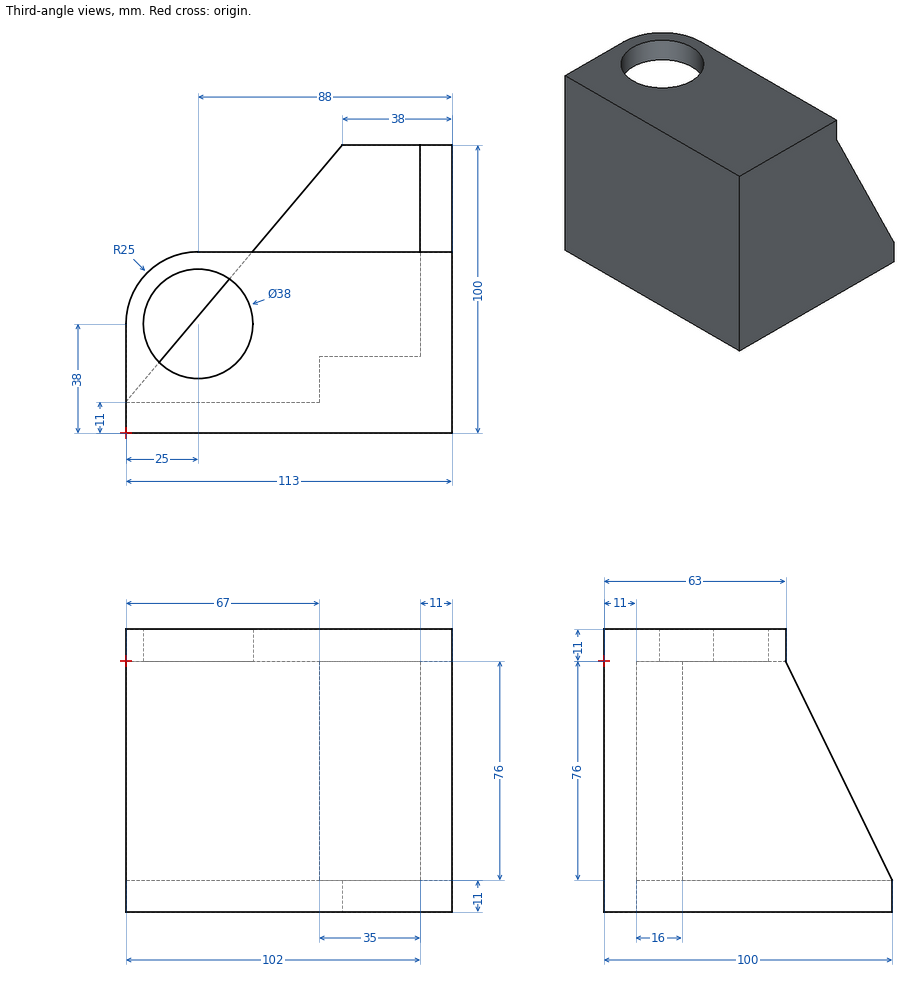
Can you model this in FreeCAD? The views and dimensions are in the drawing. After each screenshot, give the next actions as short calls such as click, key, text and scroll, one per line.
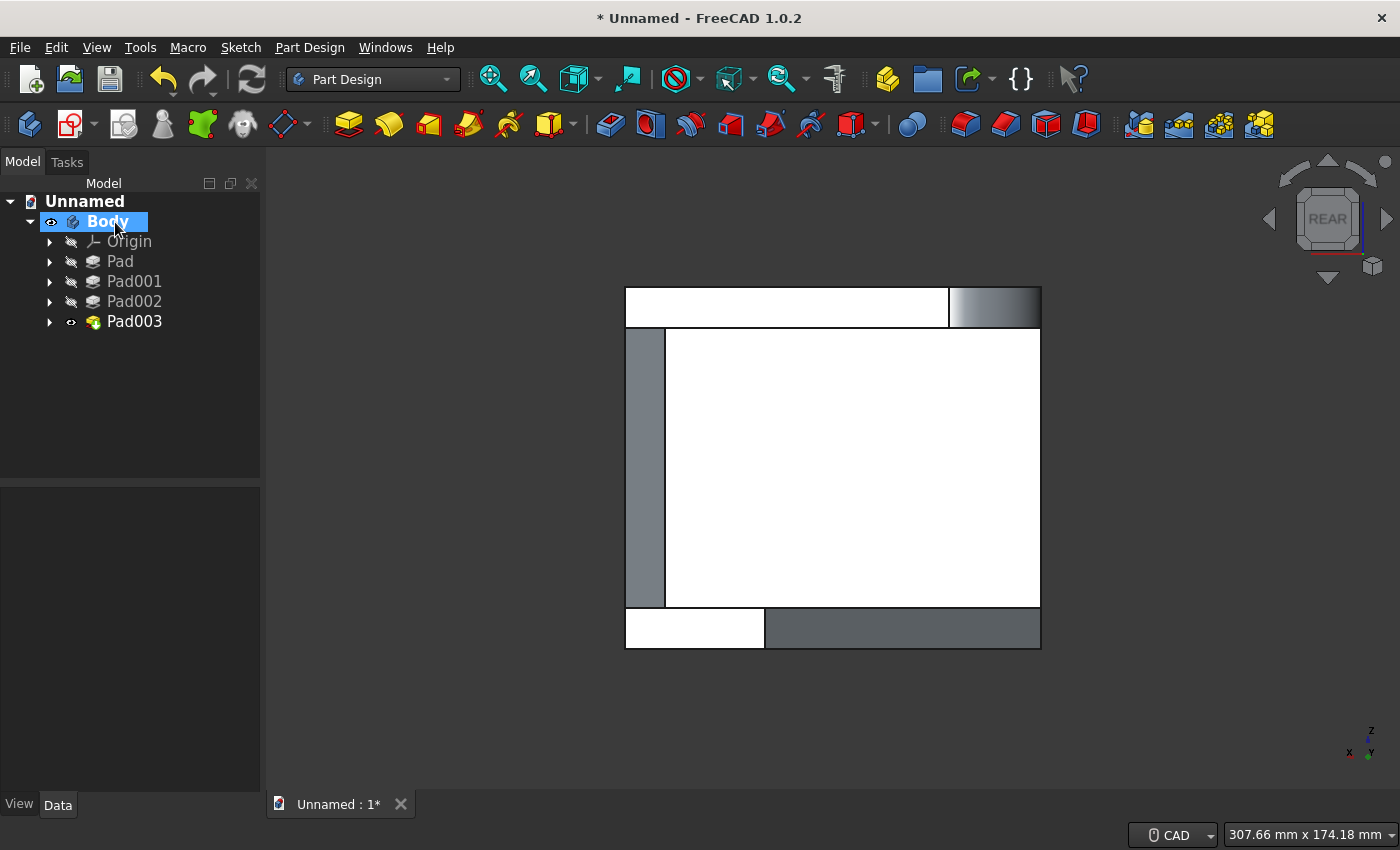
click(853, 467)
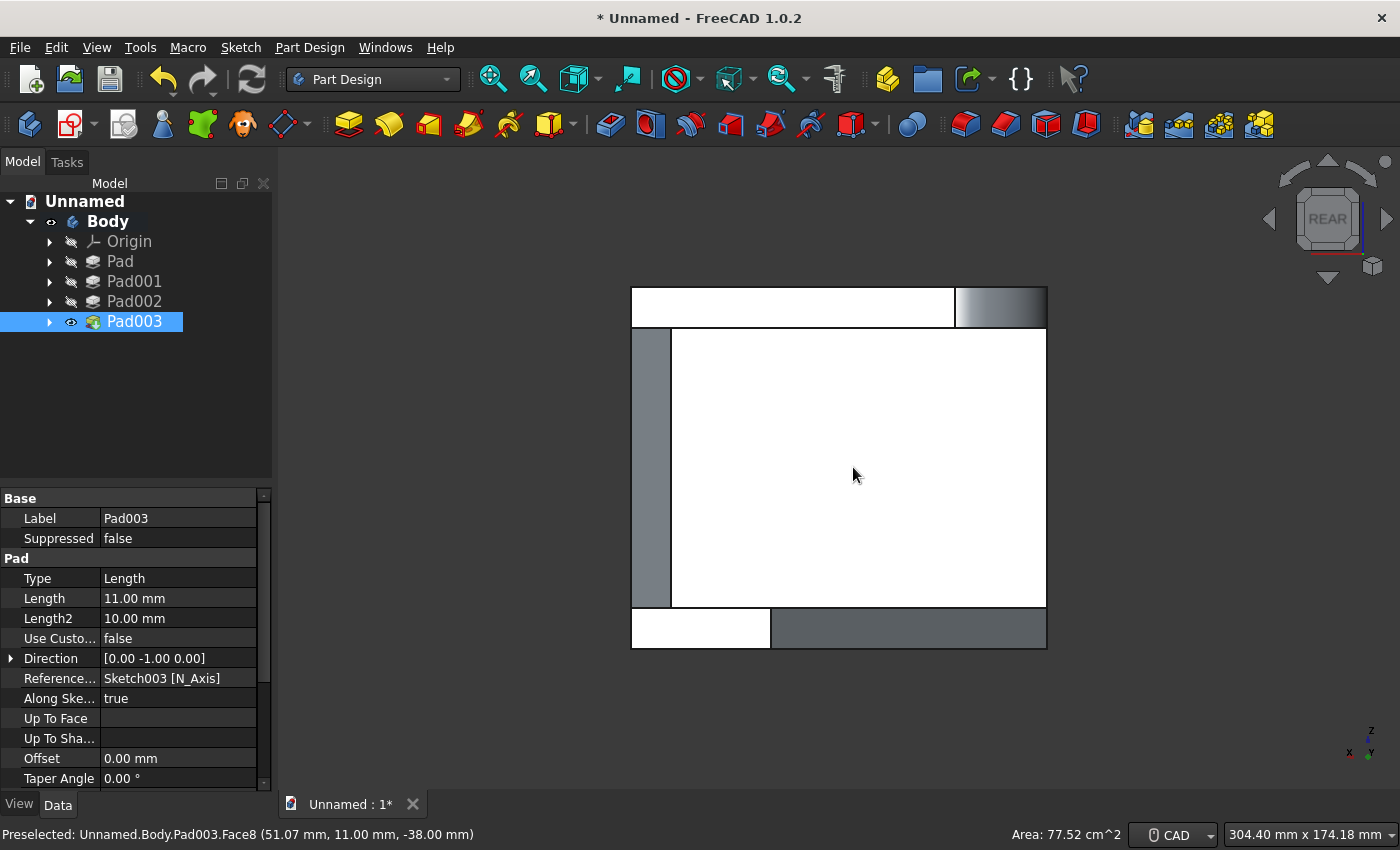
click(70, 124)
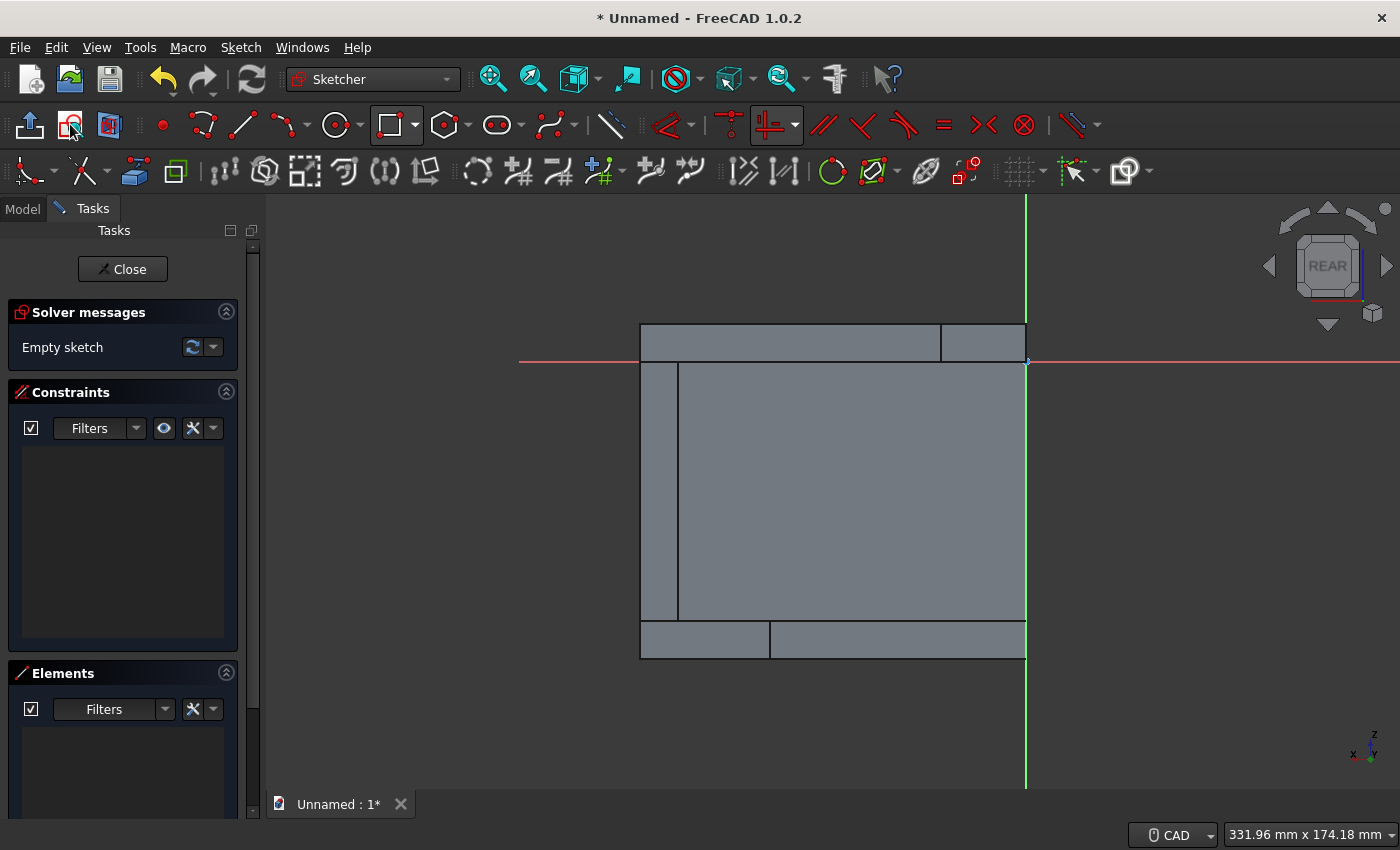
key(q)
key(s)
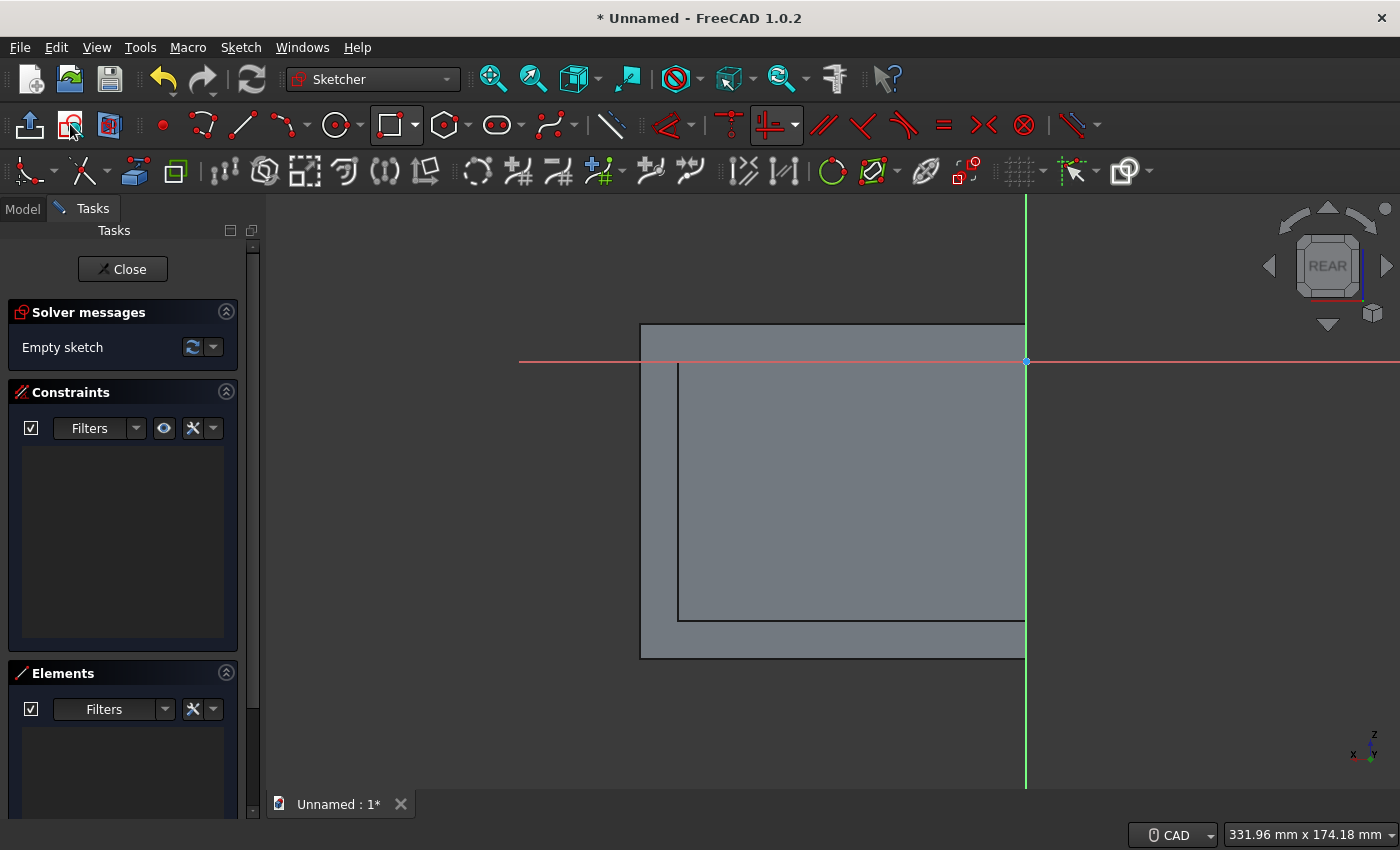
scroll(1029, 492, up, 2)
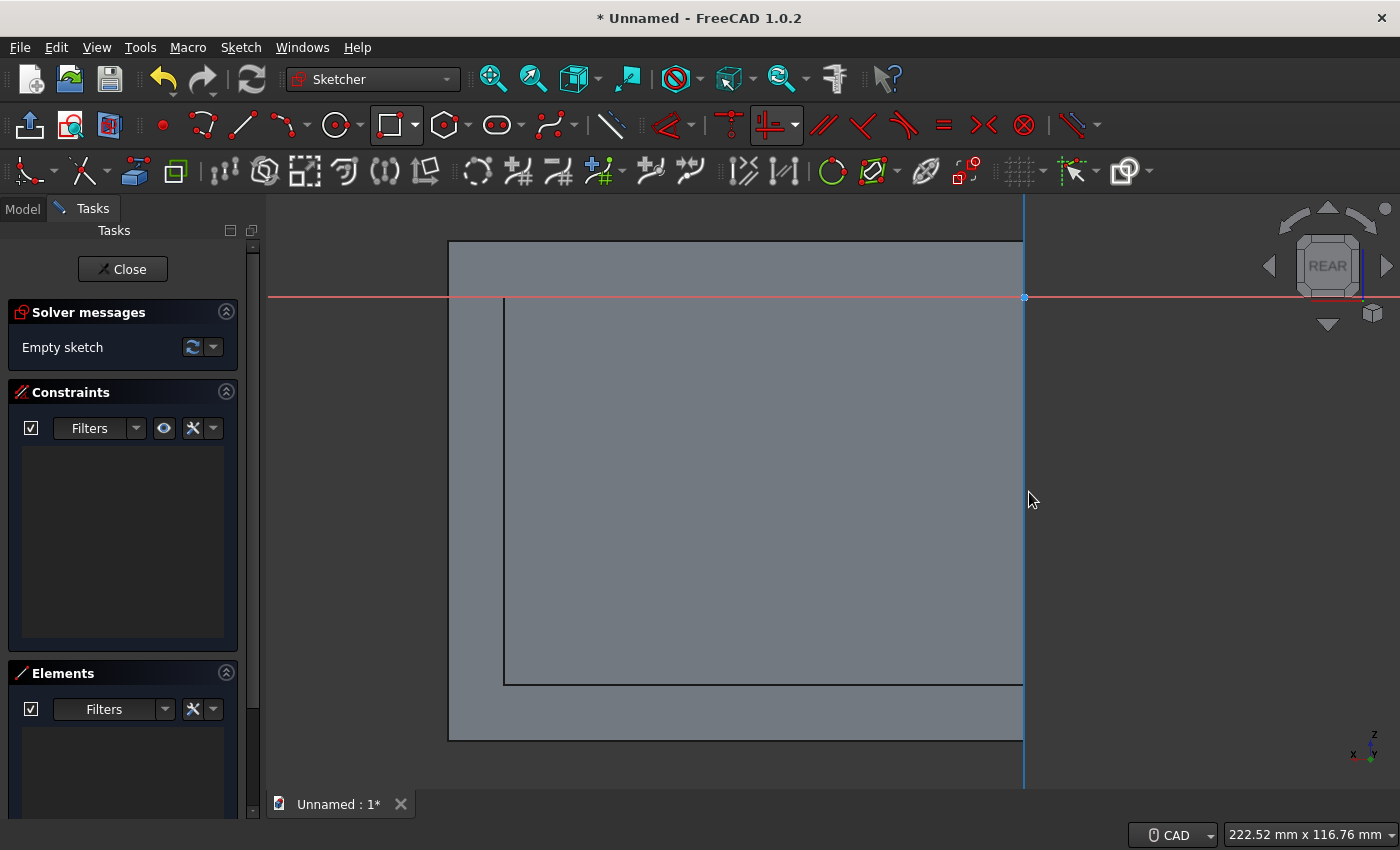
key(g)
key(r)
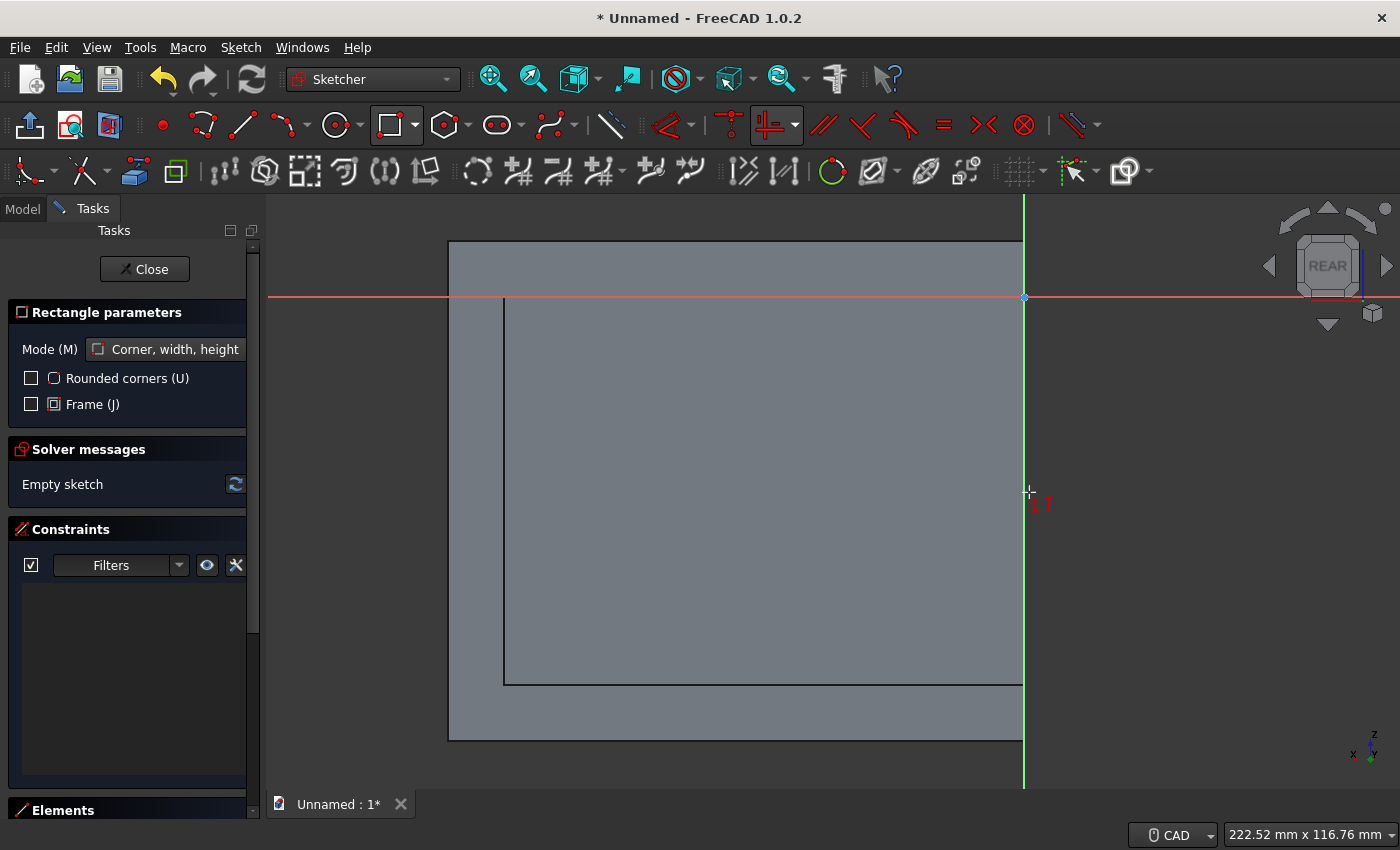
click(504, 297)
move(683, 685)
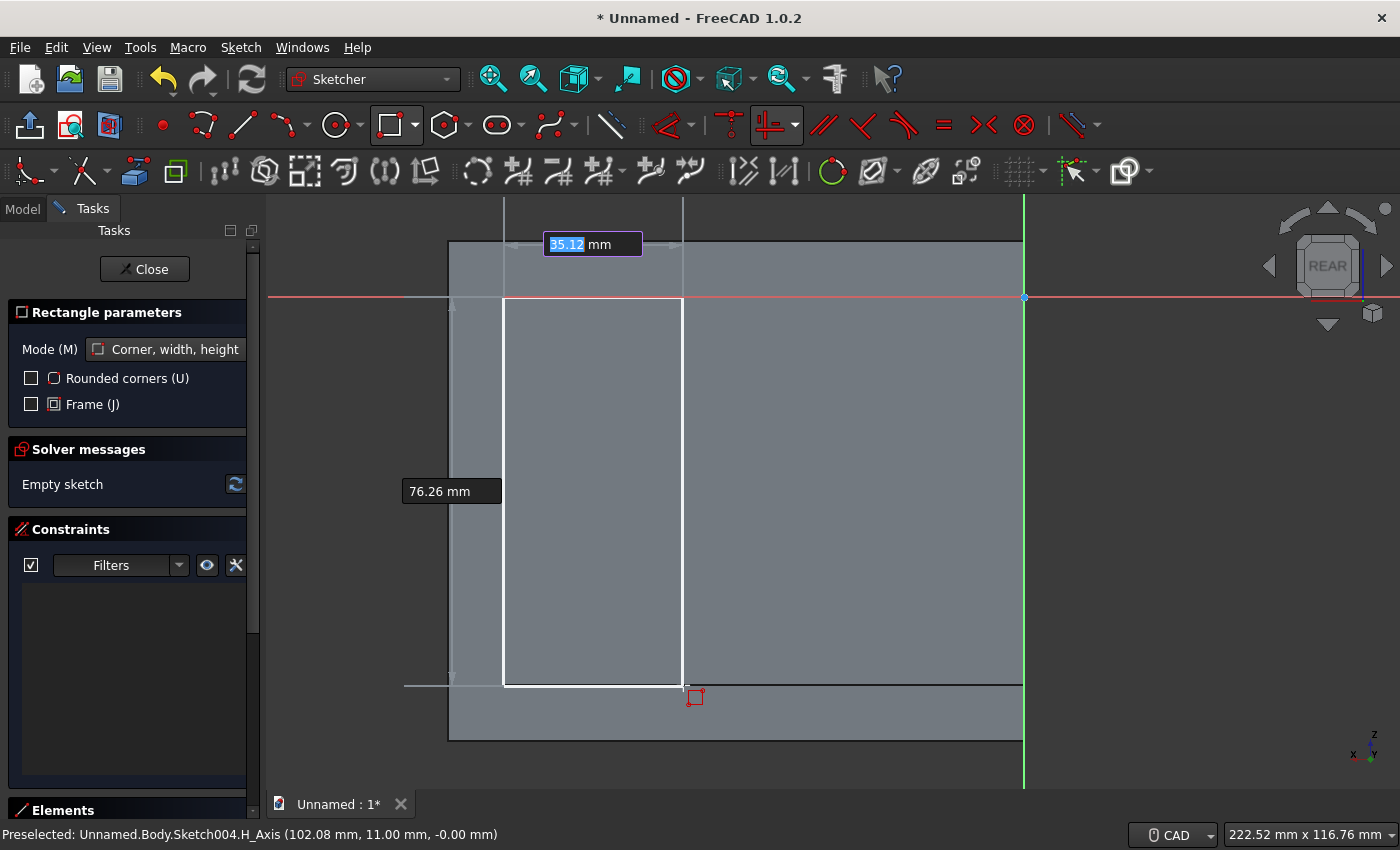
text(35)
key(Tab)
text(76)
key(Return)
key(Escape)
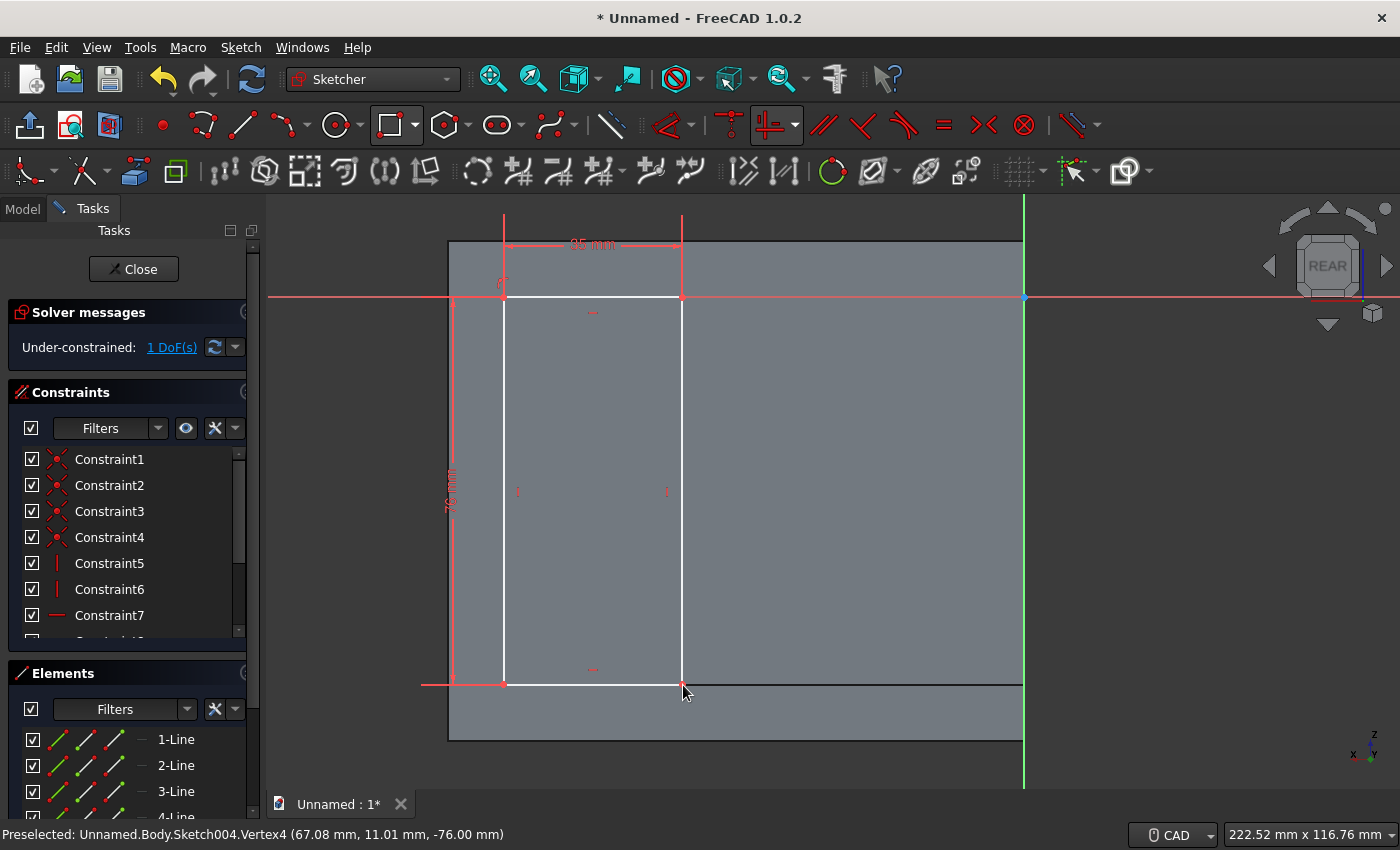
click(666, 126)